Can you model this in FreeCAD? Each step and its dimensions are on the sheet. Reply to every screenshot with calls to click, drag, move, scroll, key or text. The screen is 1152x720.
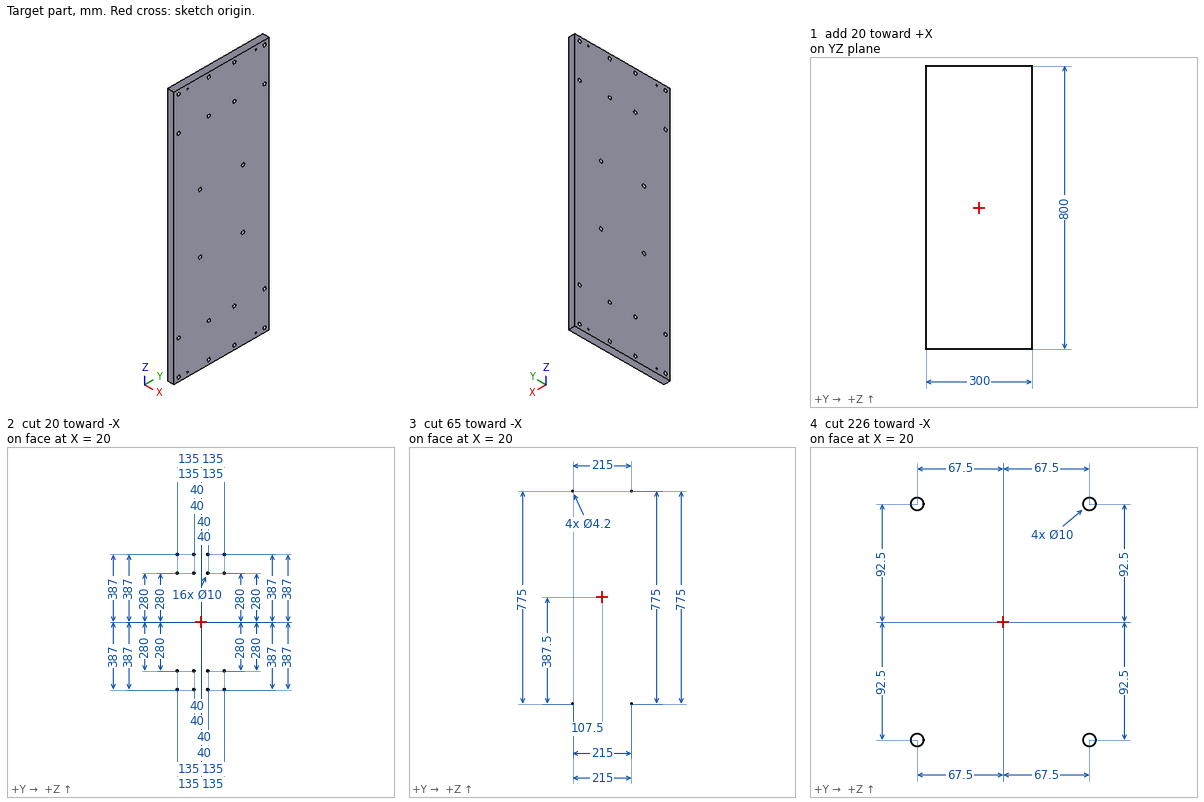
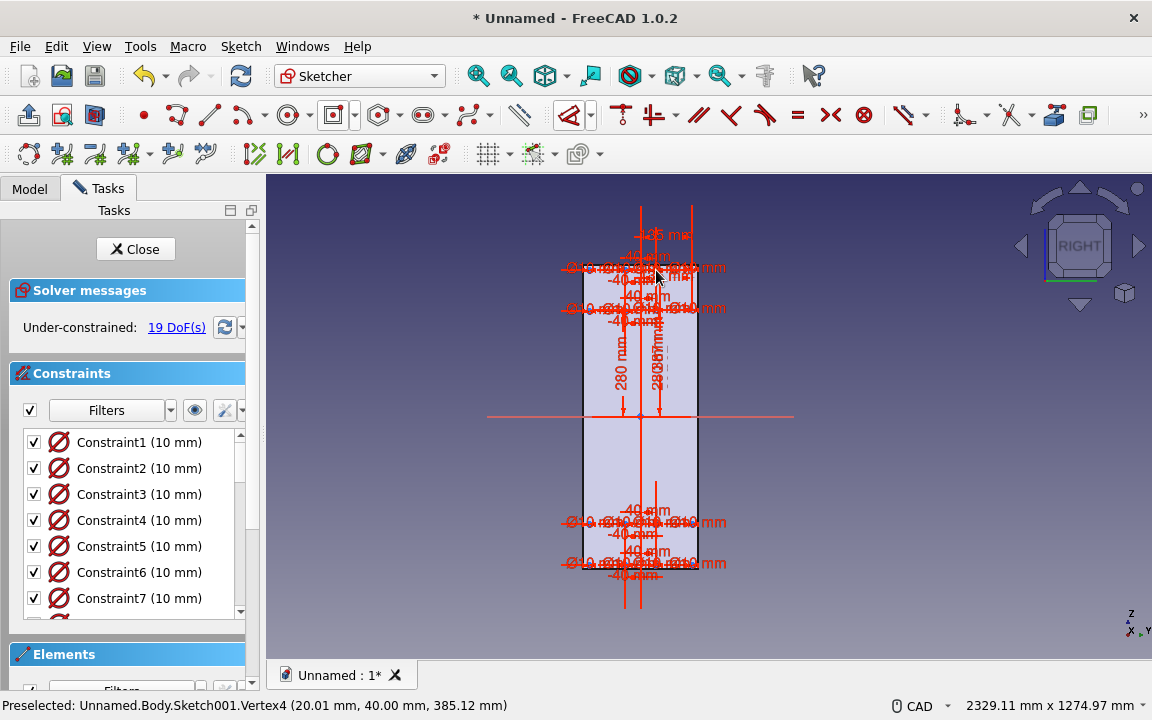
key(i)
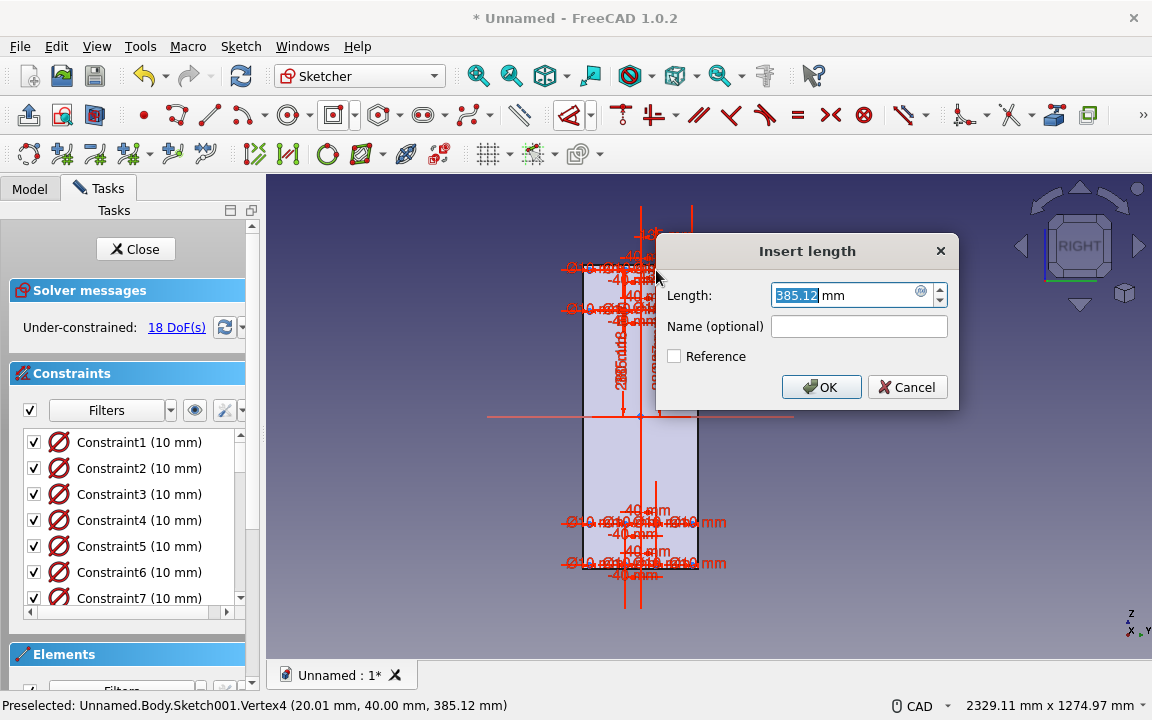
text(387)
key(Return)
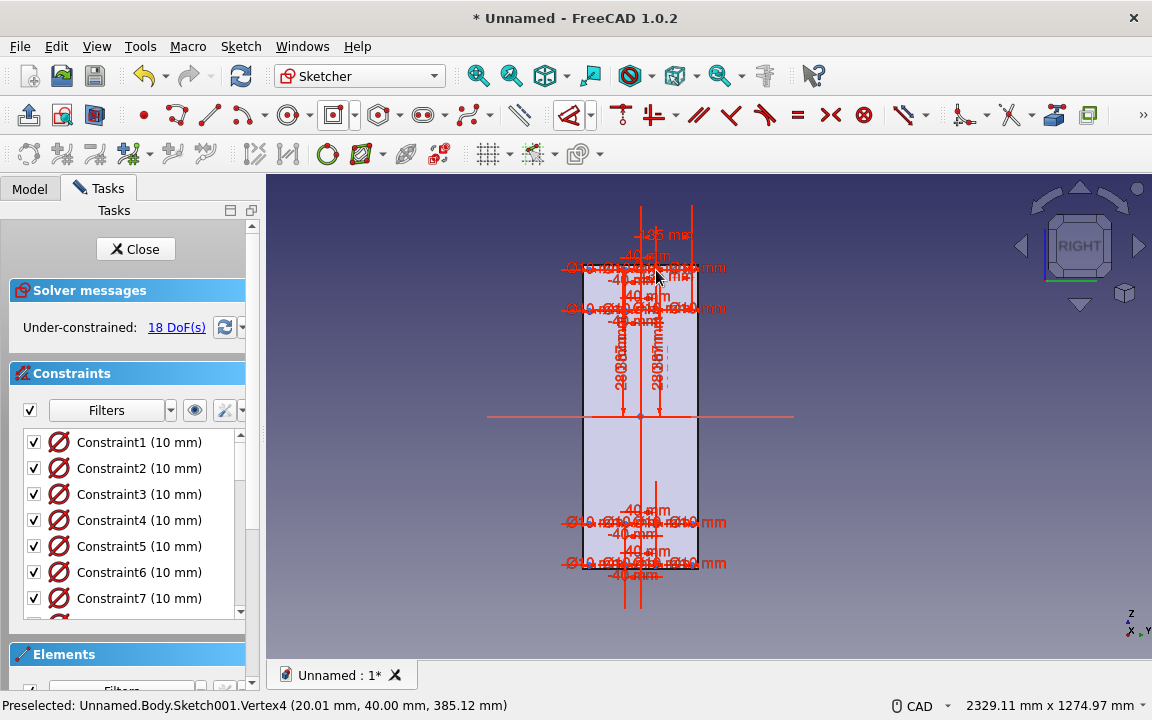
click(625, 311)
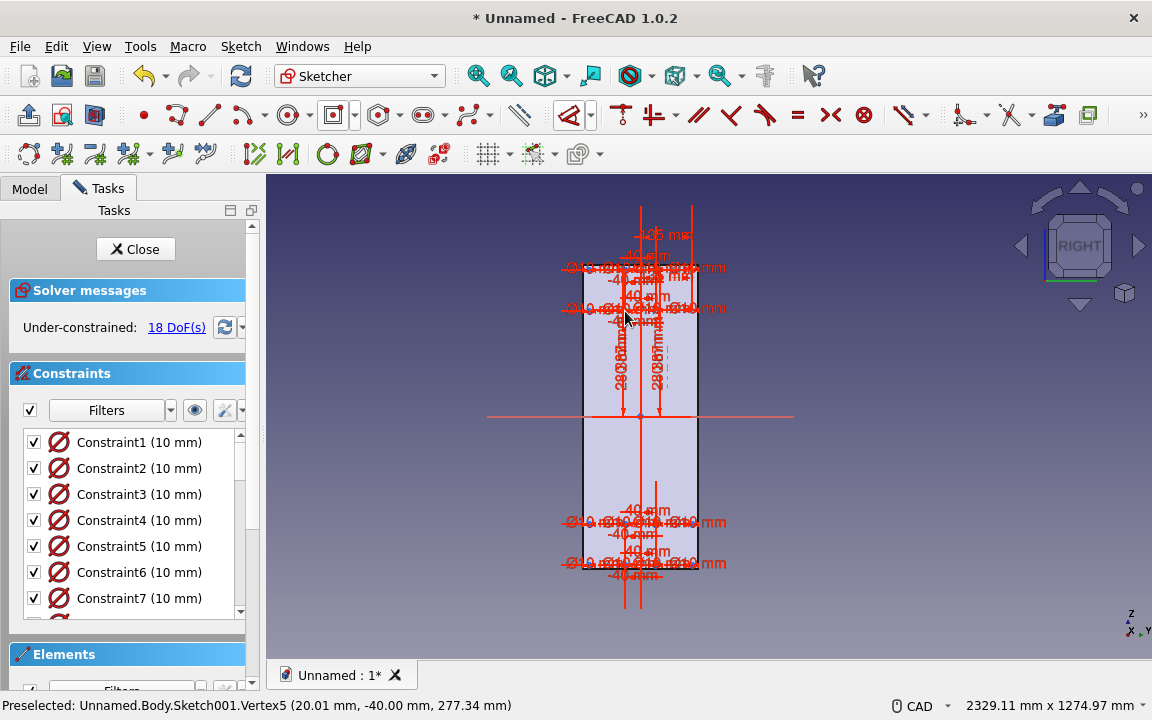
key(i)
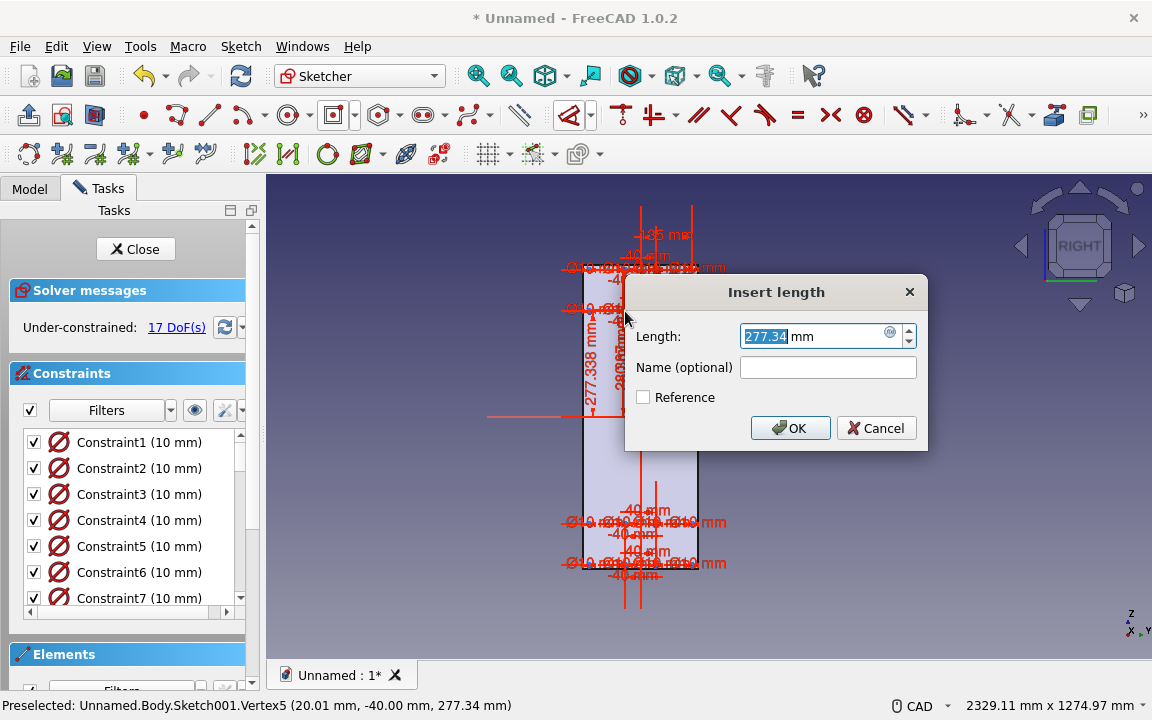
text(280)
key(Return)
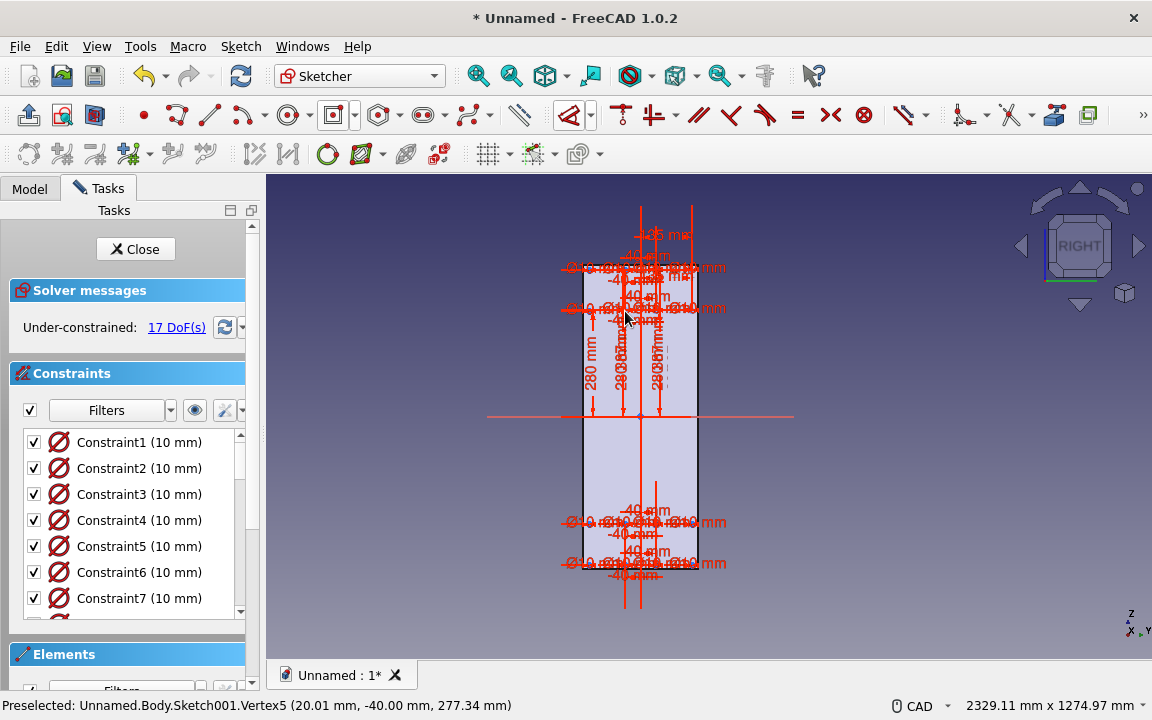
click(589, 311)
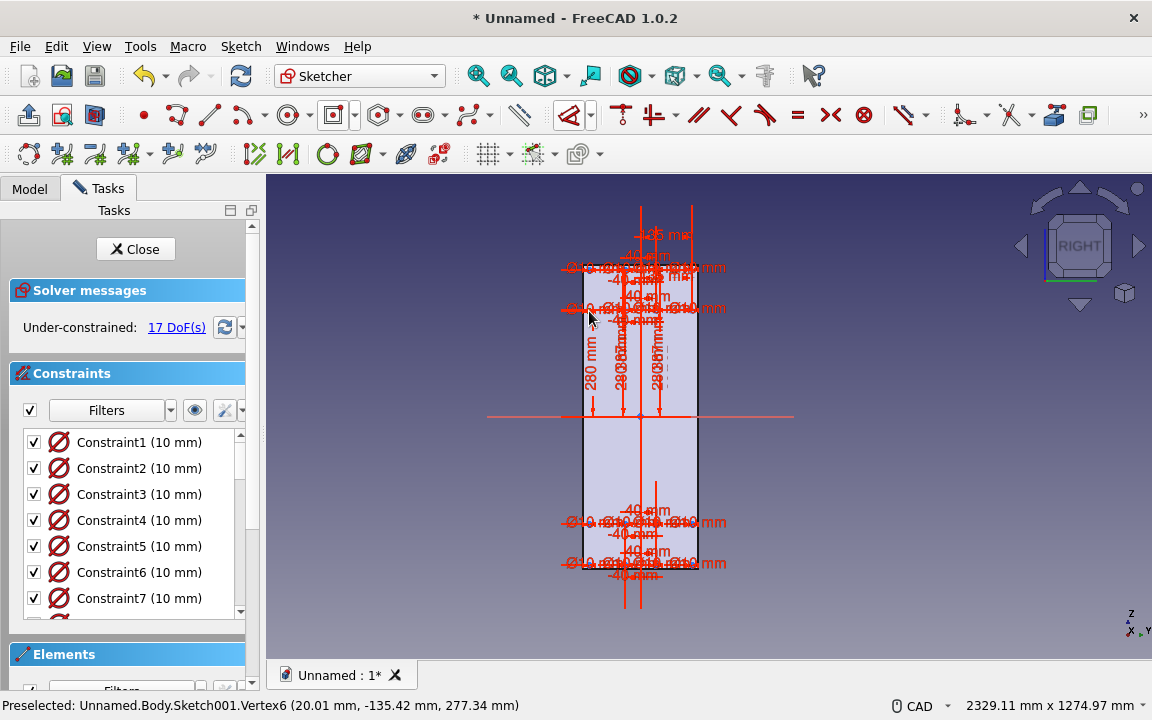
key(l)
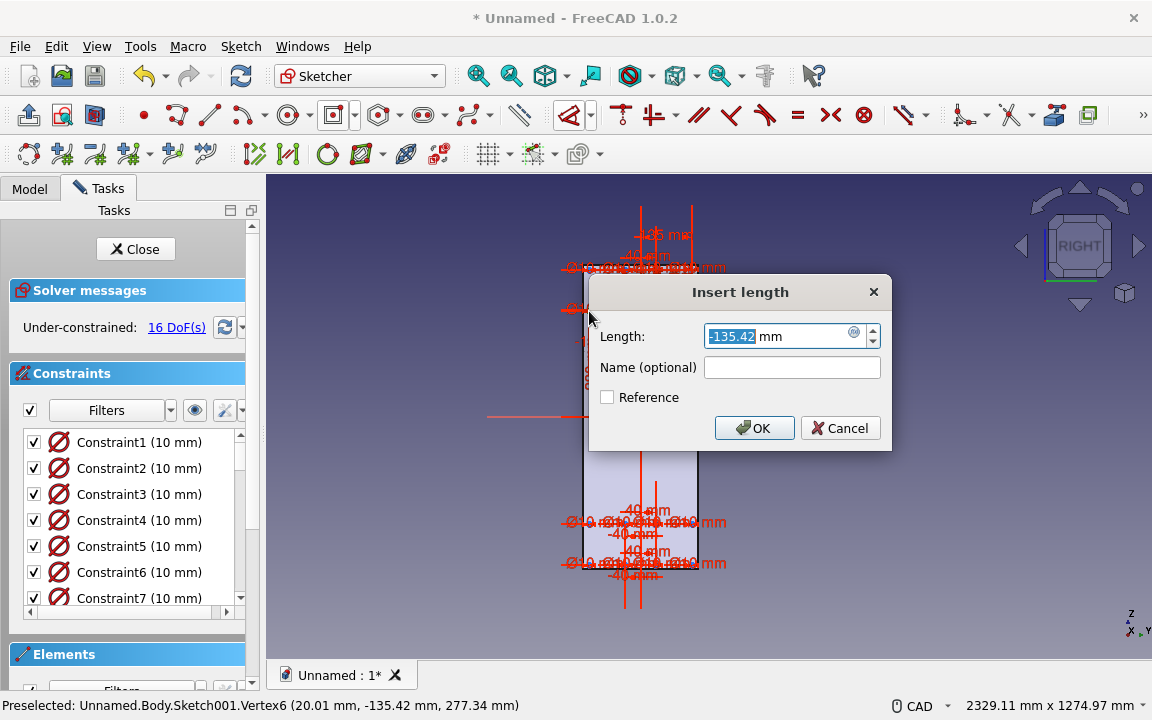
text(-135)
key(Return)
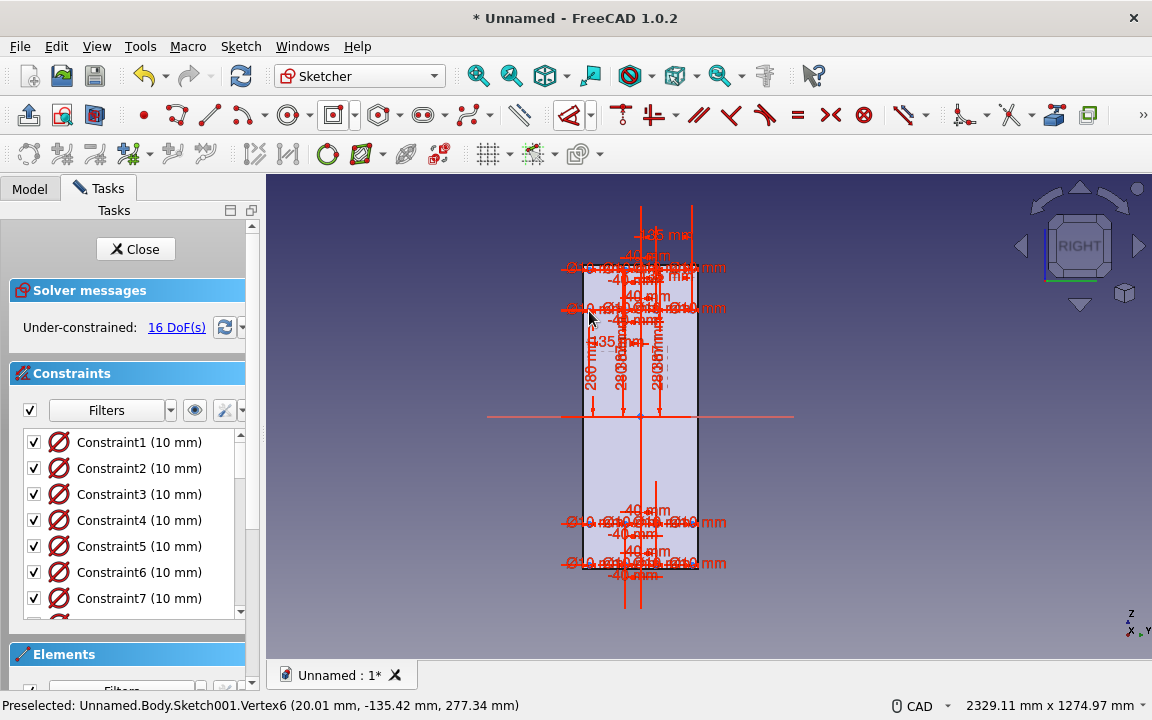
click(589, 311)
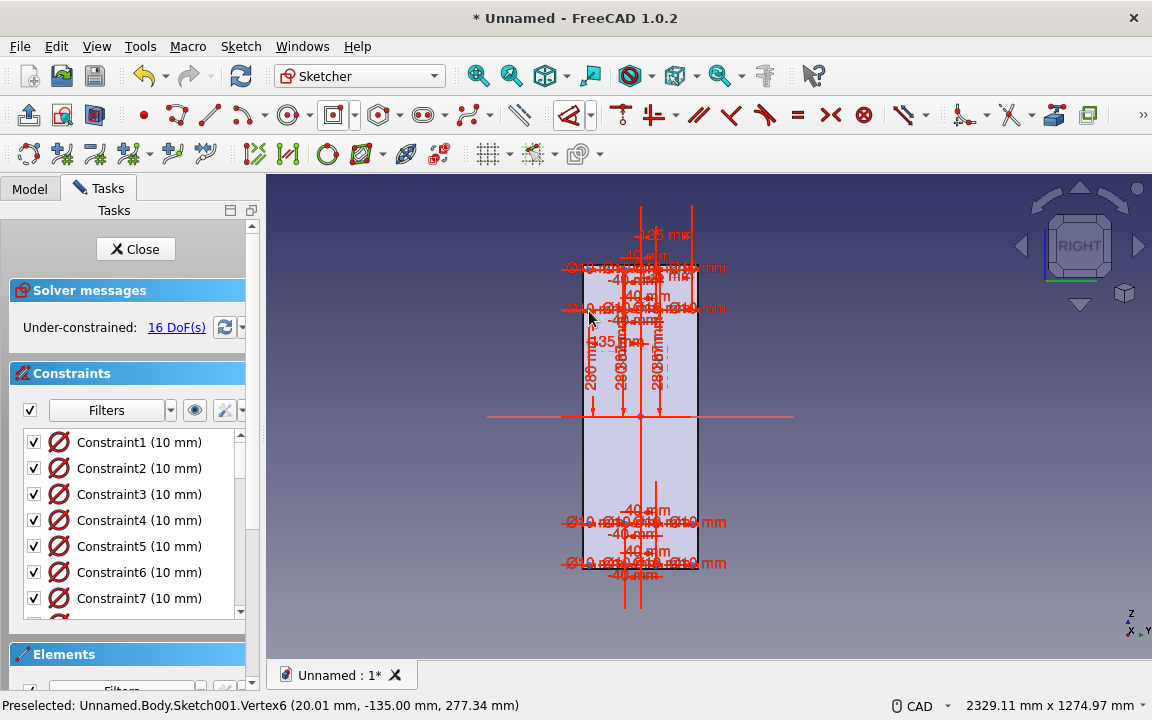
key(i)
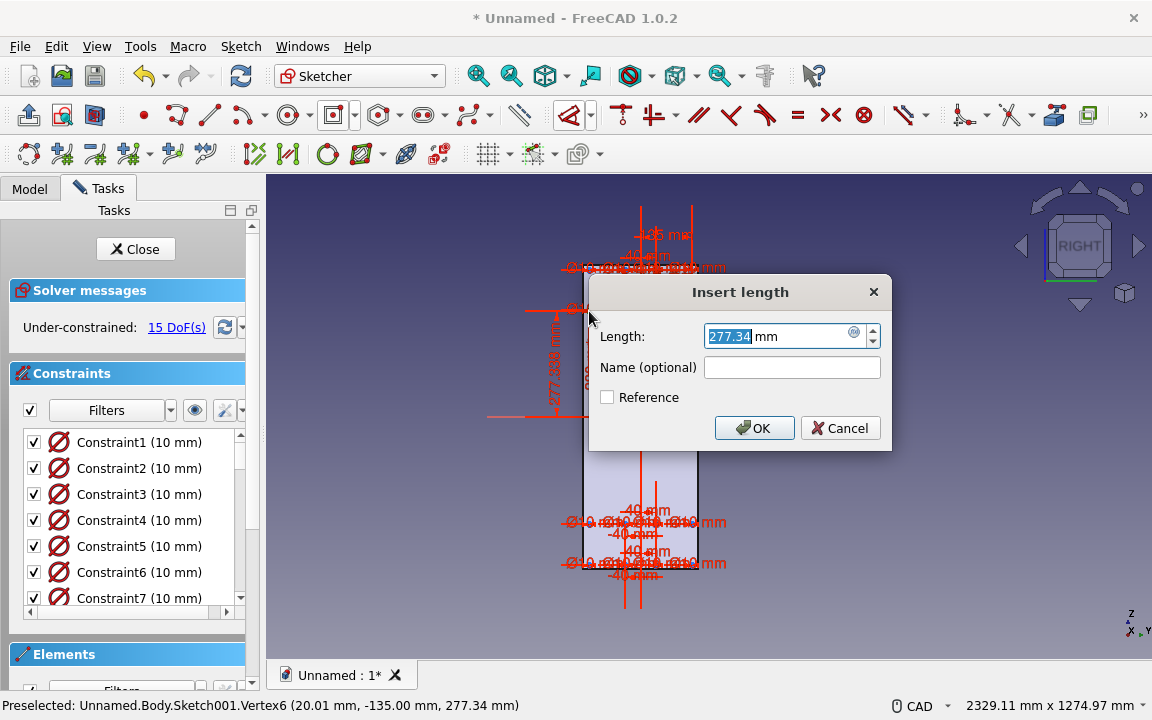
text(280)
key(Return)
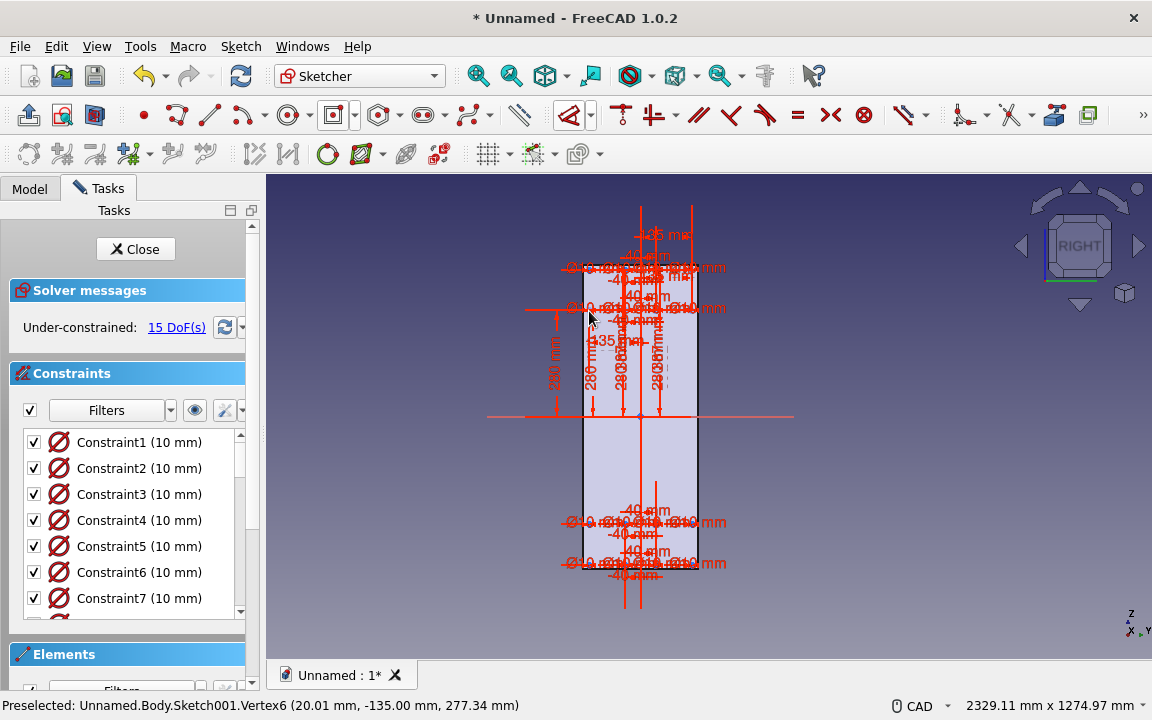
click(589, 270)